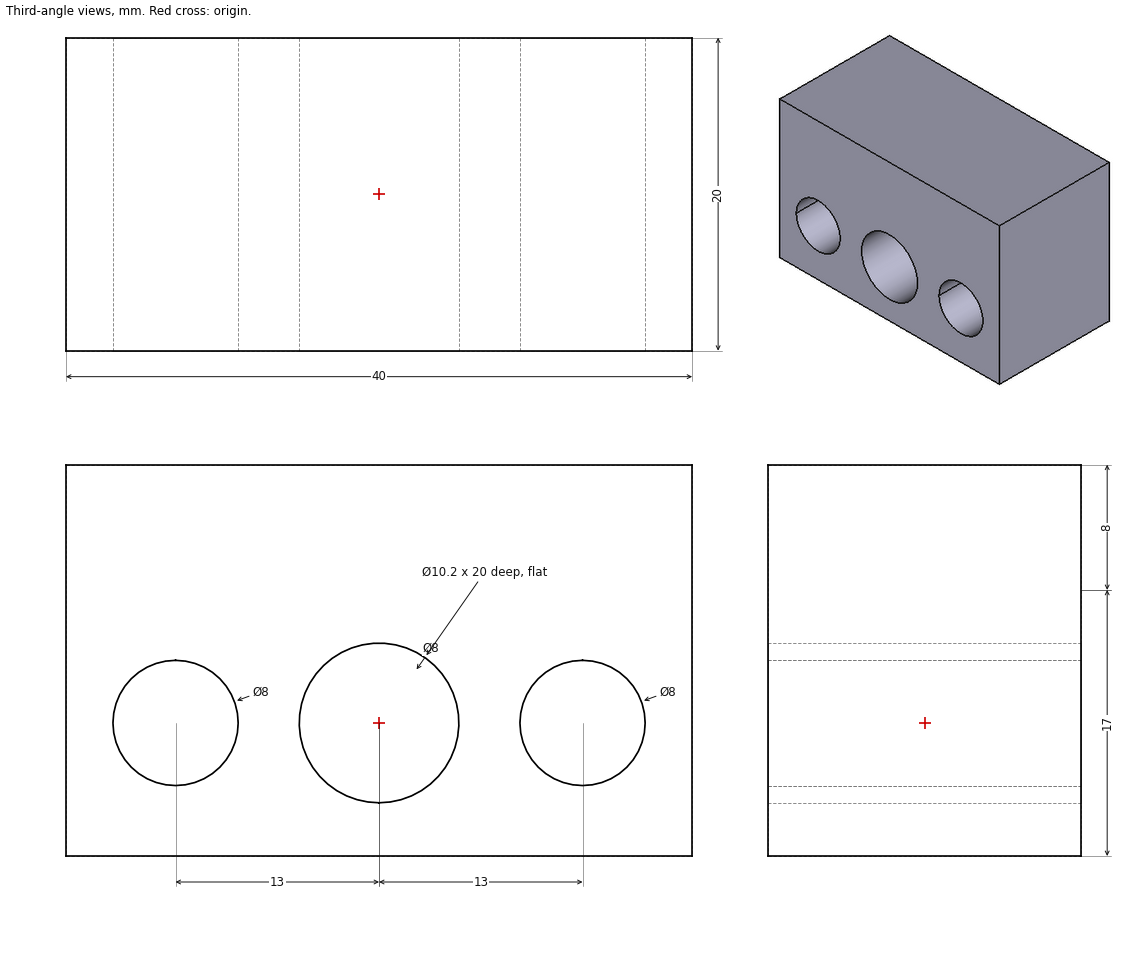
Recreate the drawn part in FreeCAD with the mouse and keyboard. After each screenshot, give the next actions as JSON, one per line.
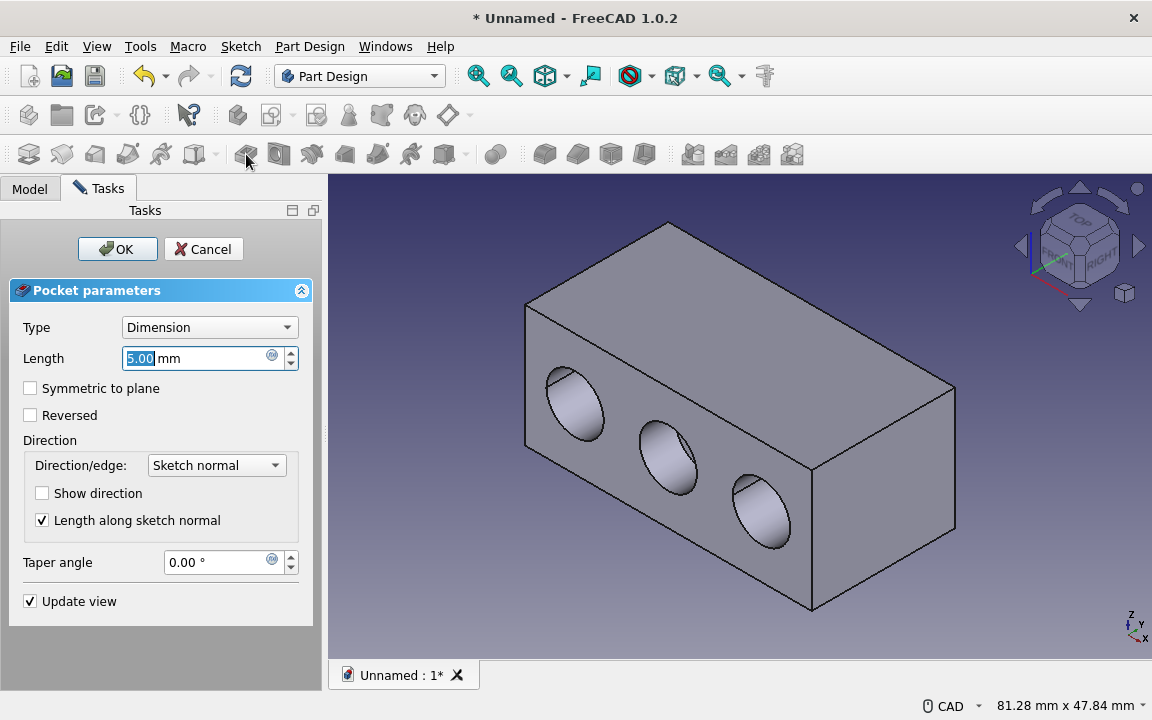
{"action": "left_click", "coordinate": [210, 328]}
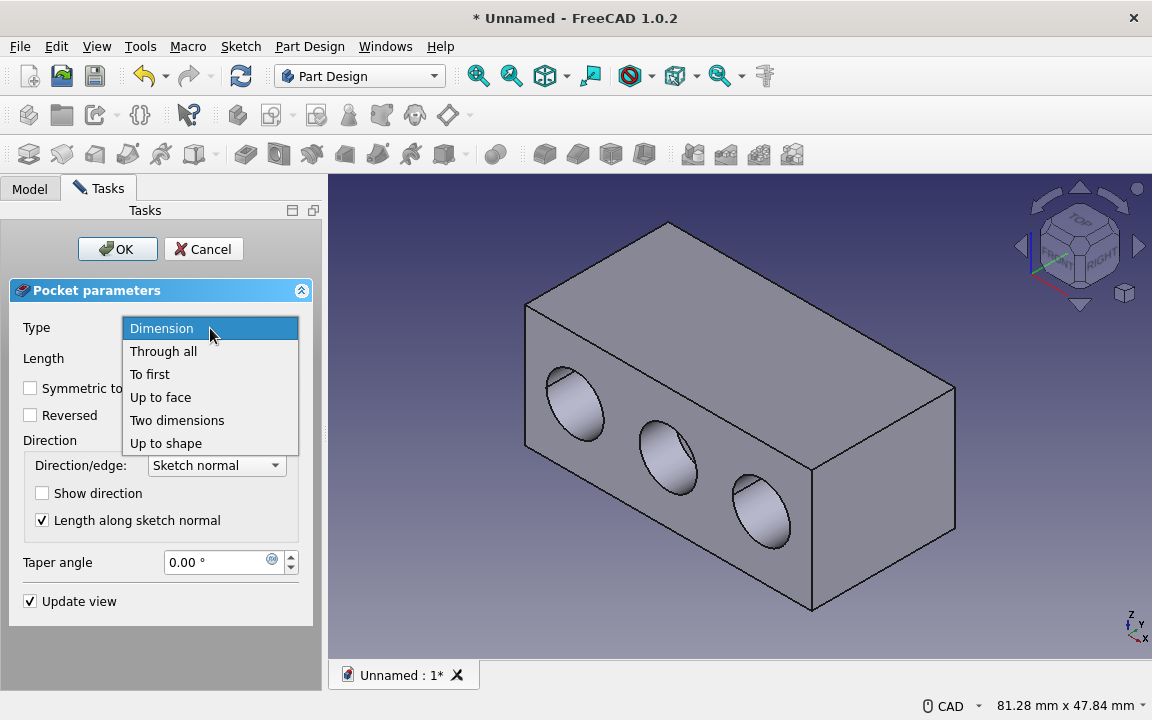
{"action": "left_click", "coordinate": [208, 374]}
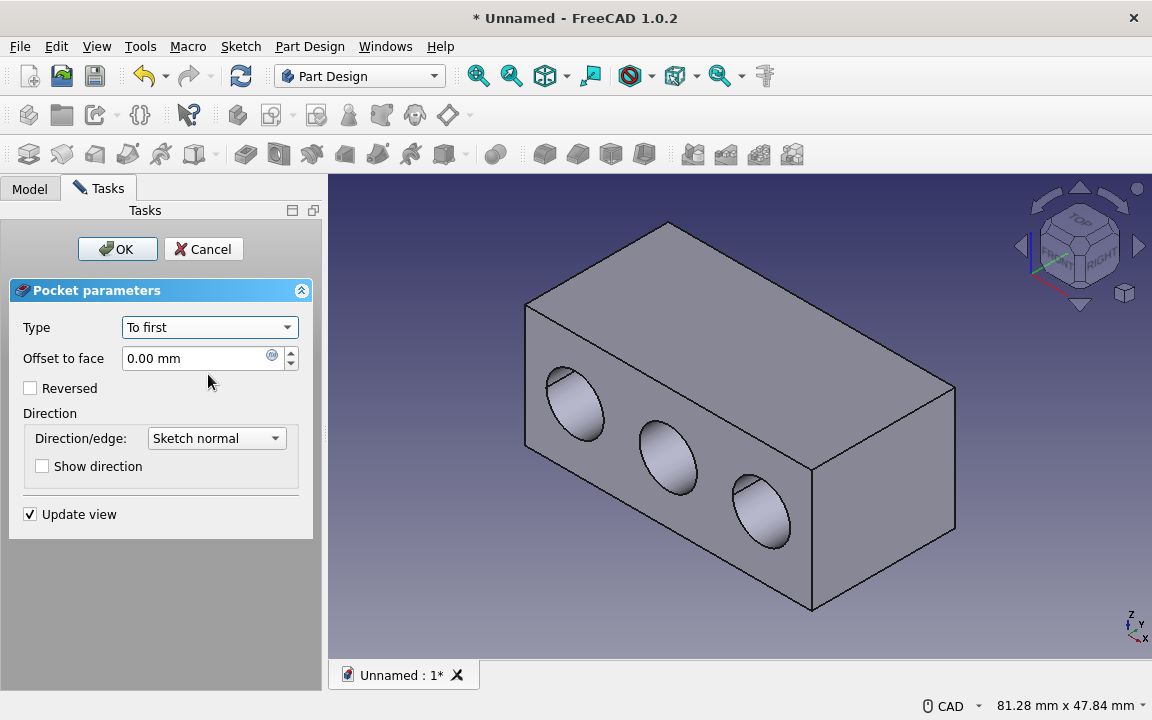
{"action": "left_click", "coordinate": [118, 249]}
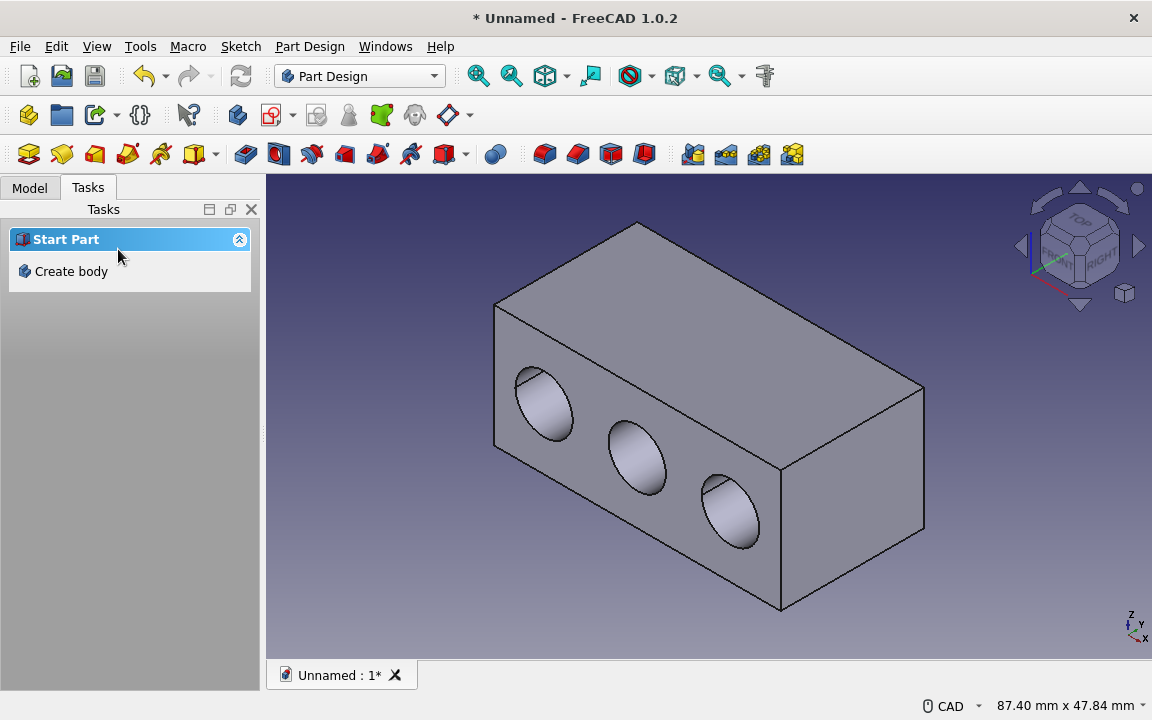
{"action": "left_click", "coordinate": [750, 369]}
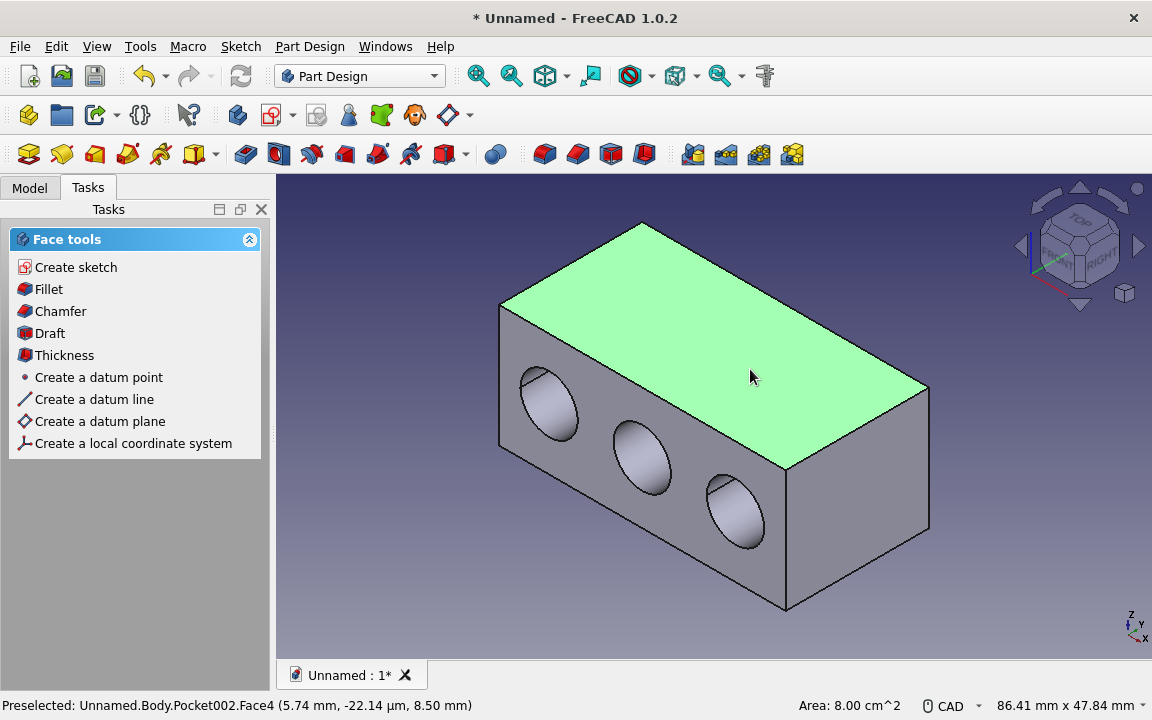
{"action": "left_click", "coordinate": [270, 116]}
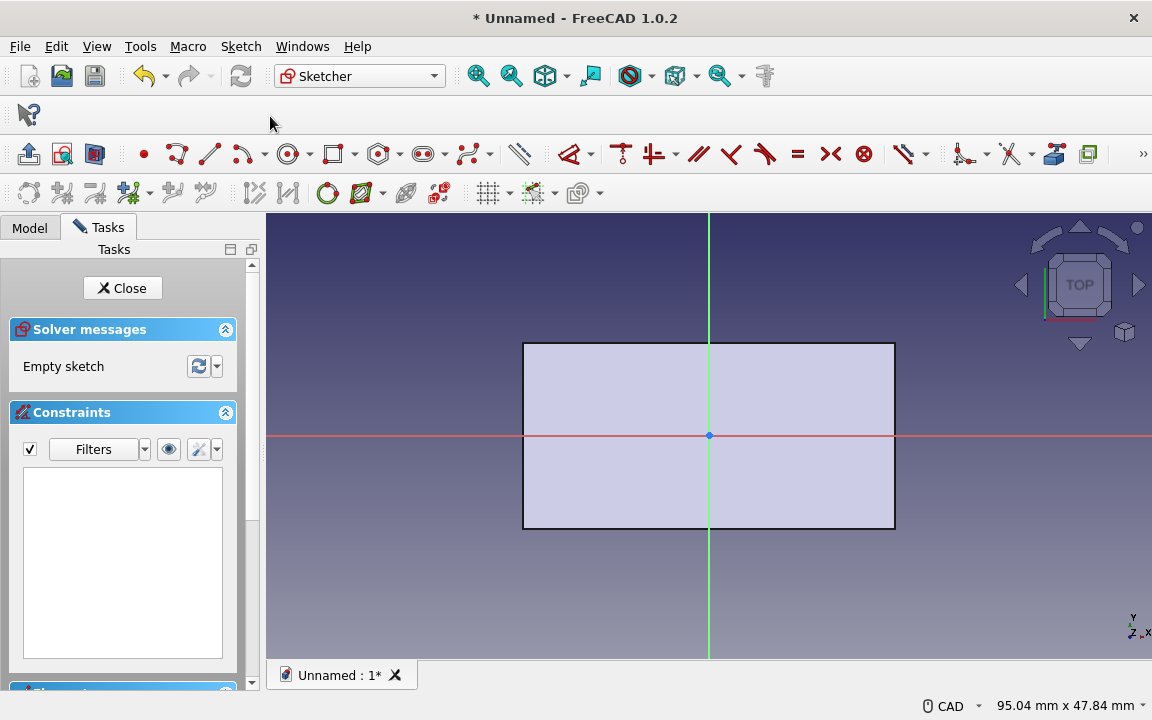
{"action": "key", "text": "g v"}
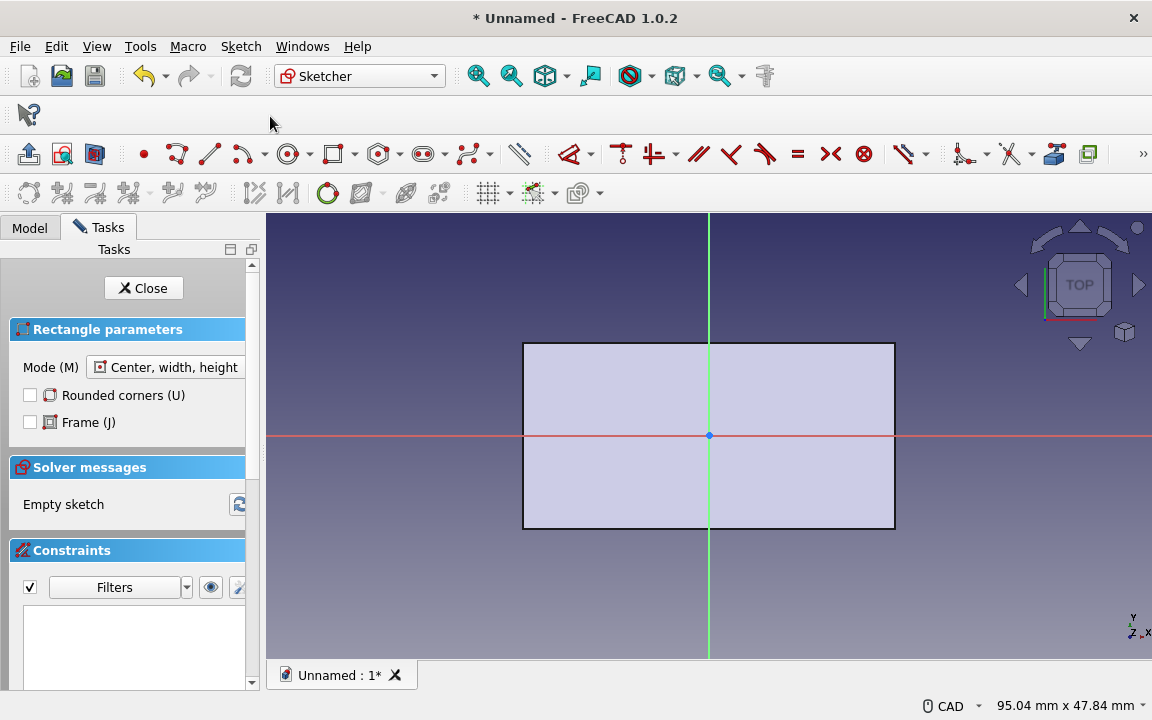
{"action": "left_click", "coordinate": [709, 436]}
{"action": "left_click", "coordinate": [895, 343]}
{"action": "key", "text": "Escape"}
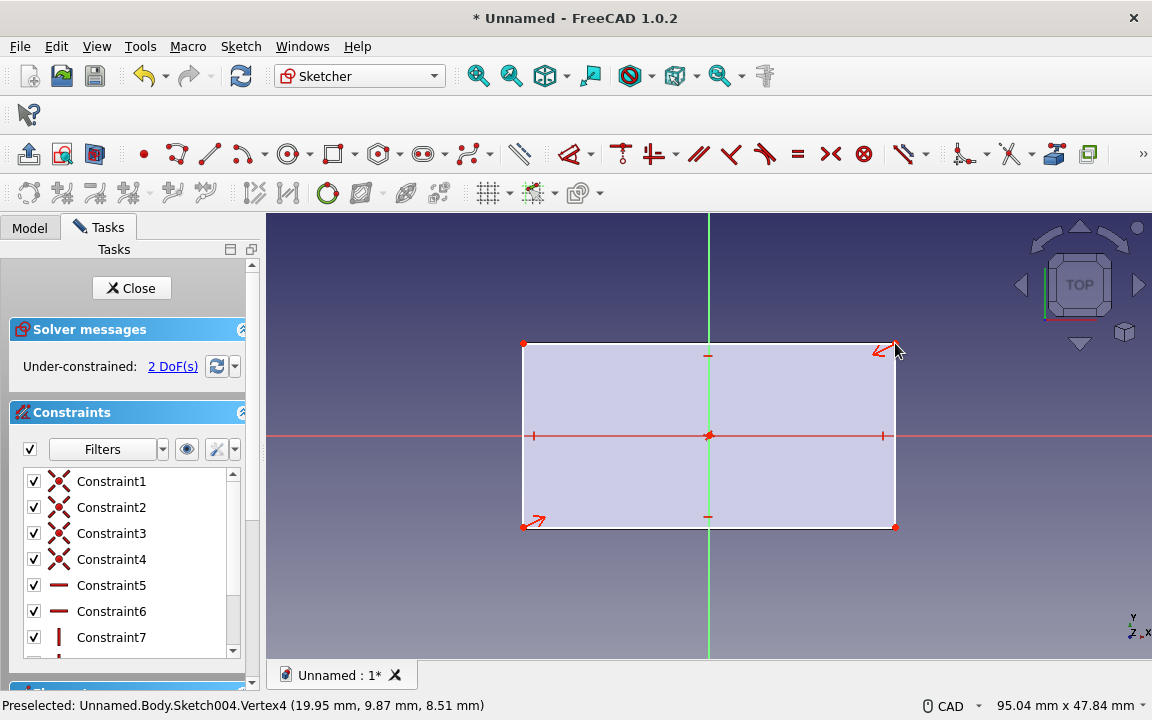
{"action": "left_click", "coordinate": [568, 154]}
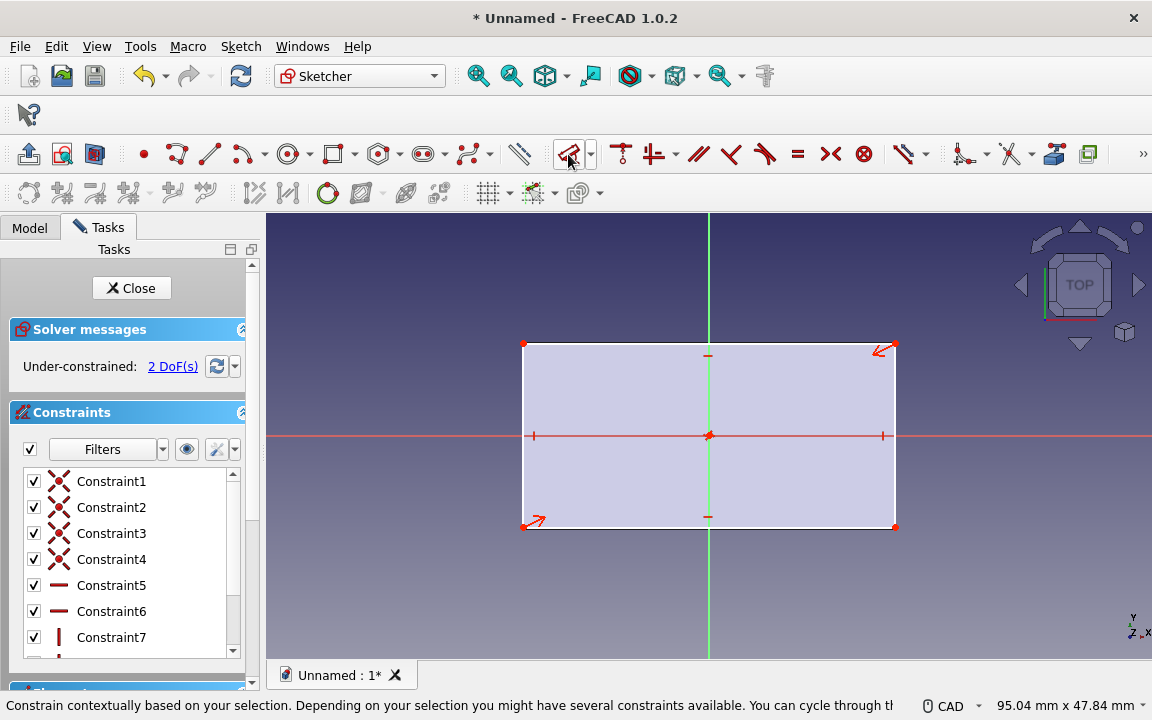
{"action": "left_click", "coordinate": [635, 528]}
{"action": "left_click", "coordinate": [623, 562]}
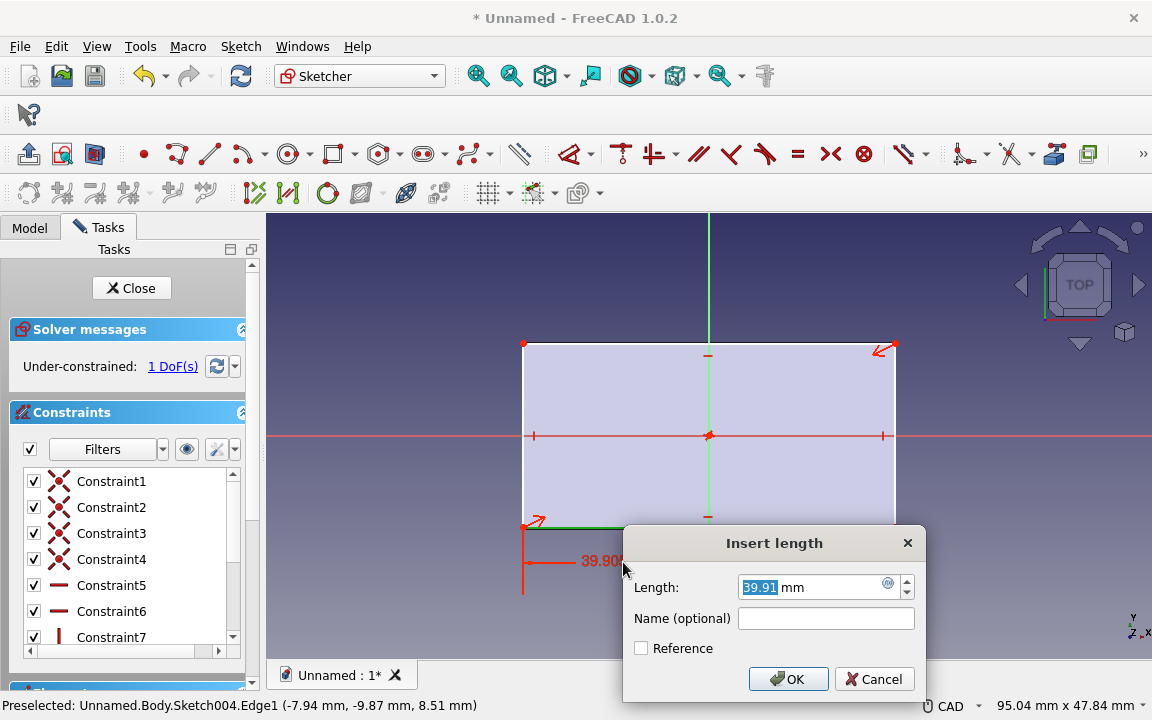
{"action": "type", "text": "40"}
{"action": "key", "text": "Return"}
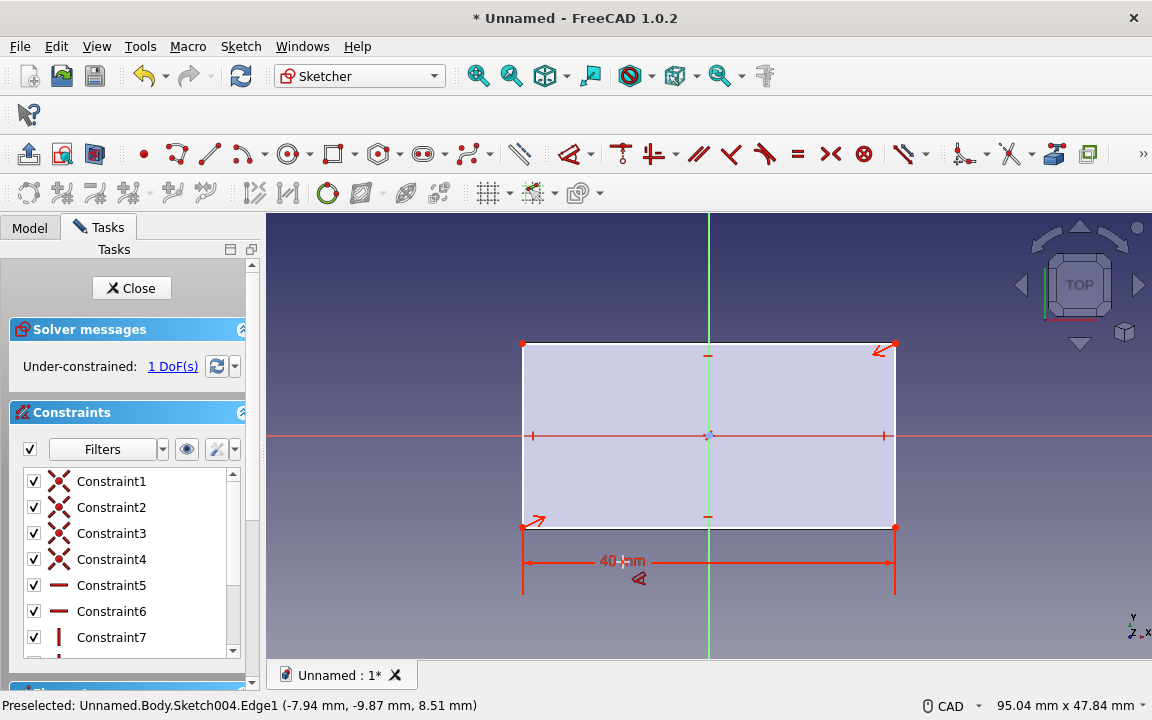
{"action": "left_click", "coordinate": [895, 473]}
{"action": "left_click", "coordinate": [929, 394]}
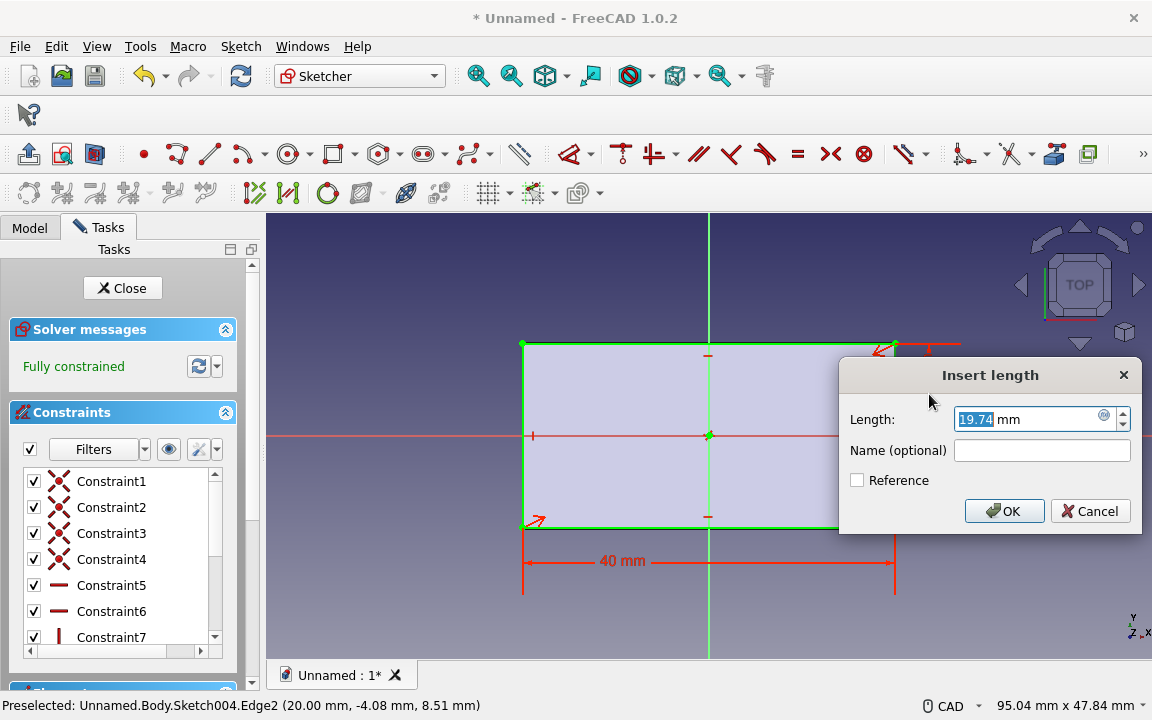
{"action": "type", "text": "20"}
{"action": "key", "text": "Return"}
{"action": "key", "text": "Escape"}